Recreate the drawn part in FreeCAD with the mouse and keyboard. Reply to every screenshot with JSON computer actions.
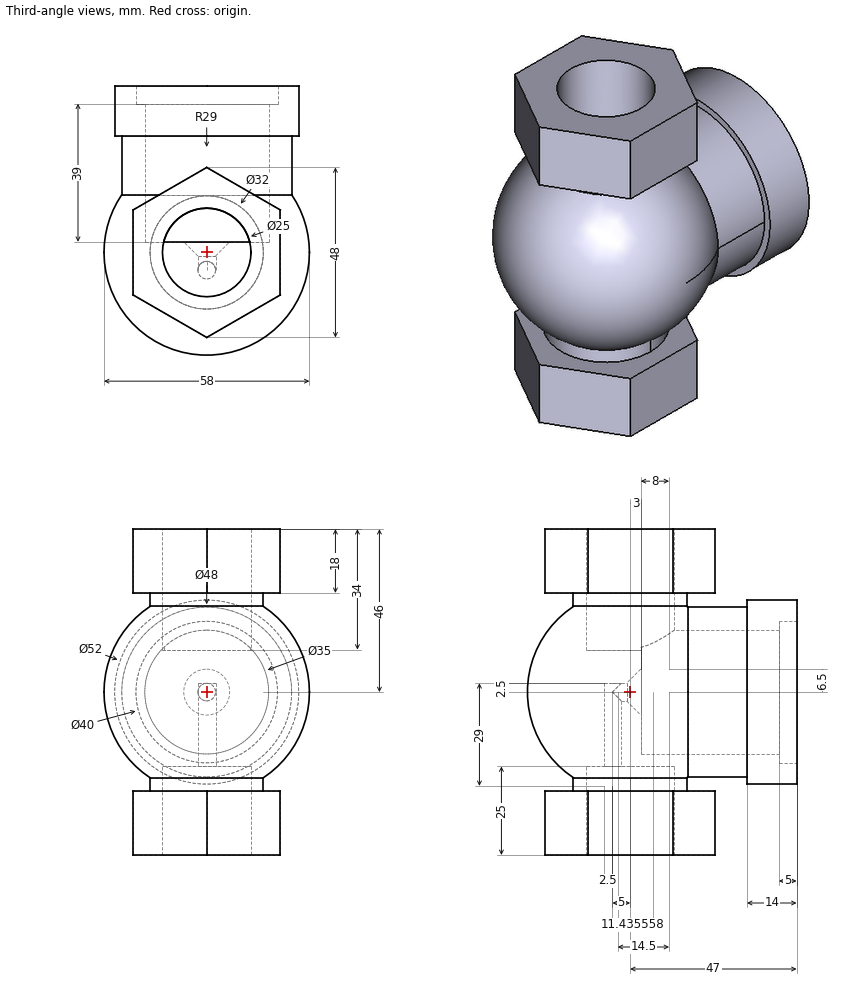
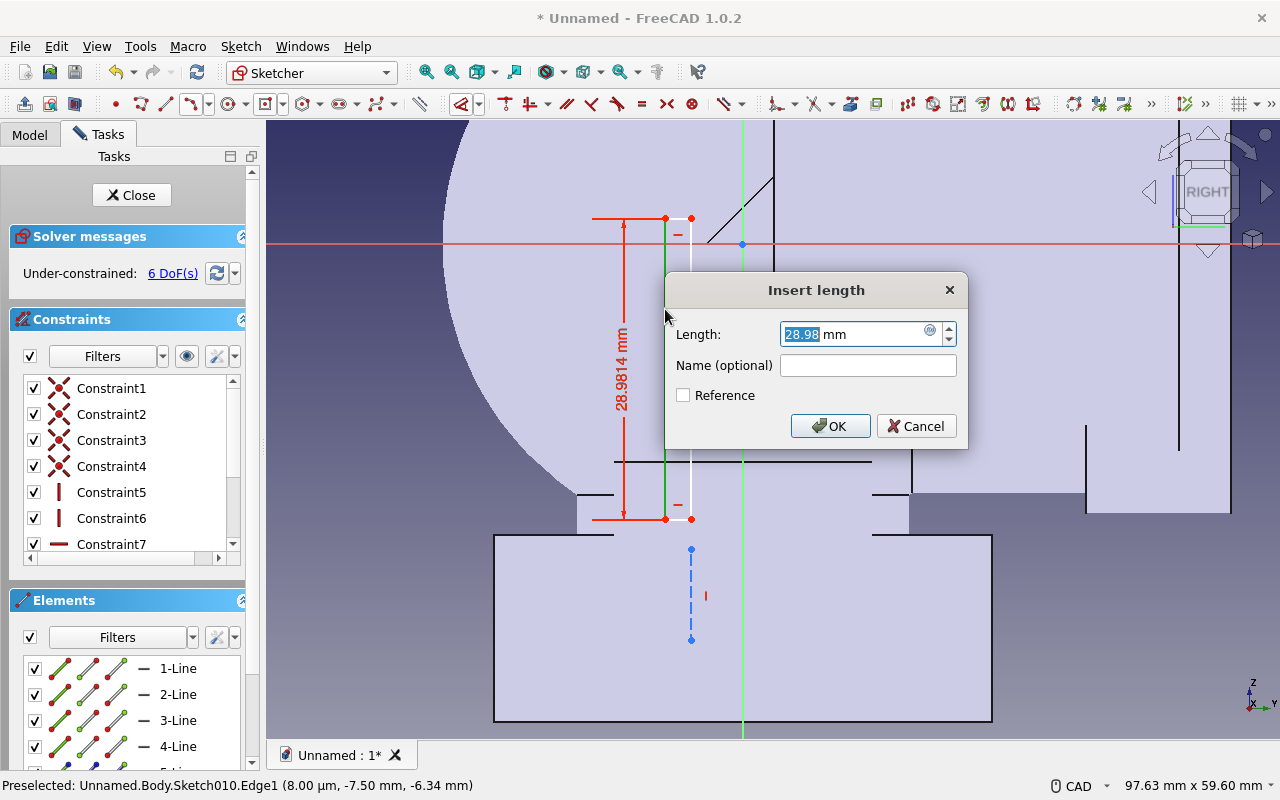
{"action": "type", "text": "29"}
{"action": "key", "text": "Return"}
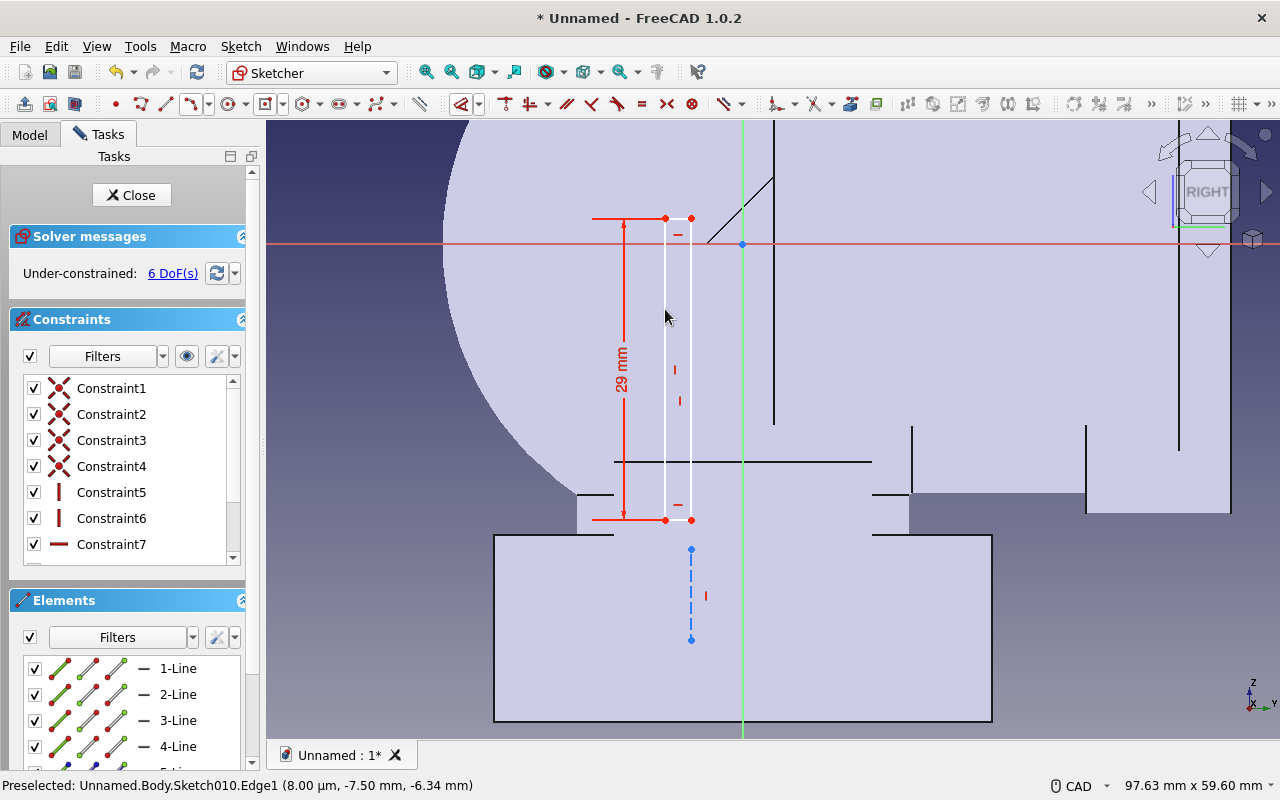
{"action": "left_click", "coordinate": [691, 520]}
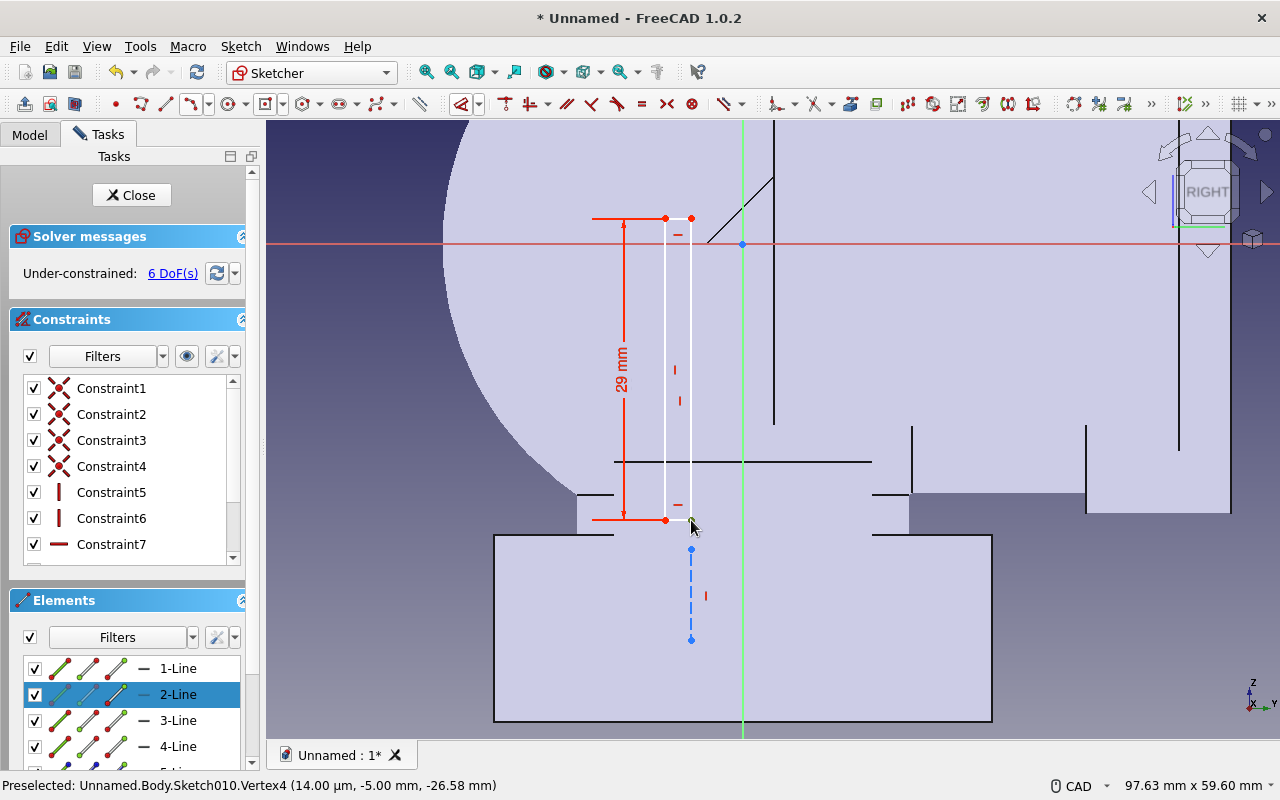
{"action": "key", "text": "l"}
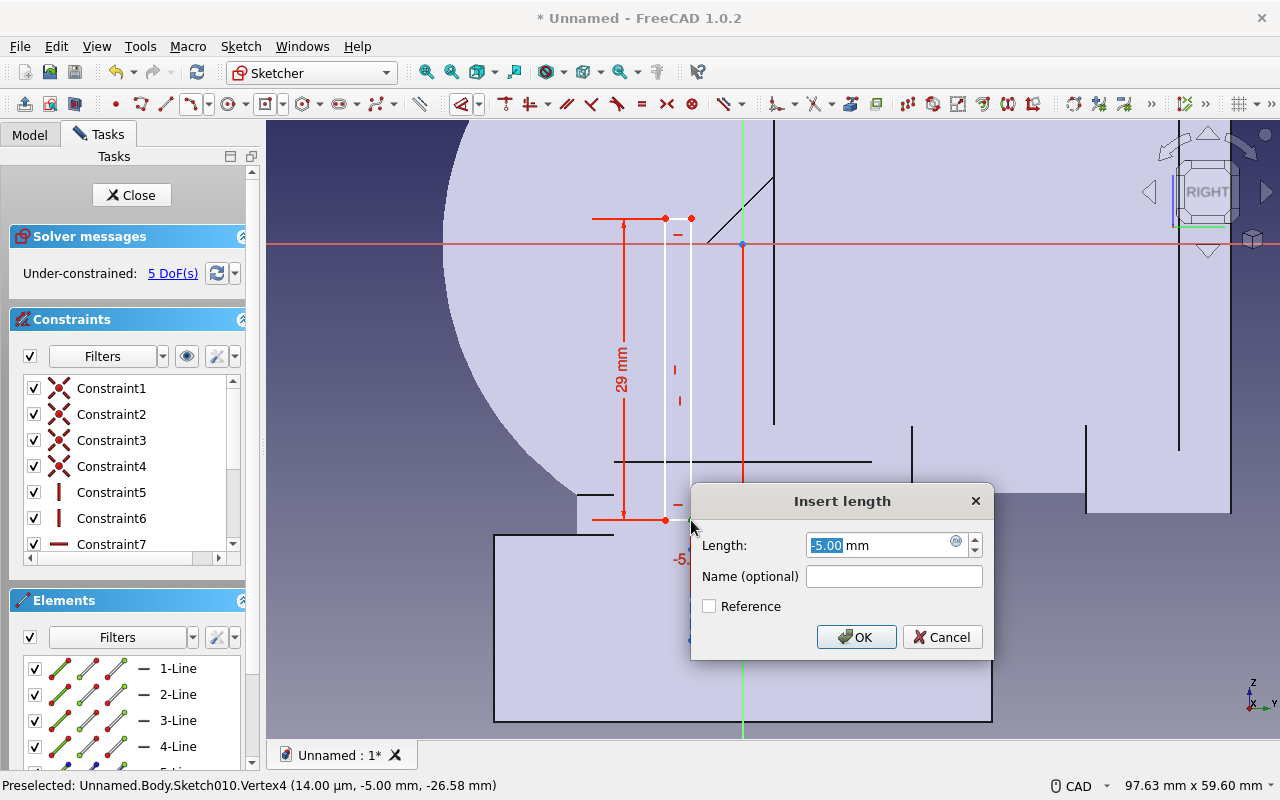
{"action": "type", "text": "-5"}
{"action": "key", "text": "Return"}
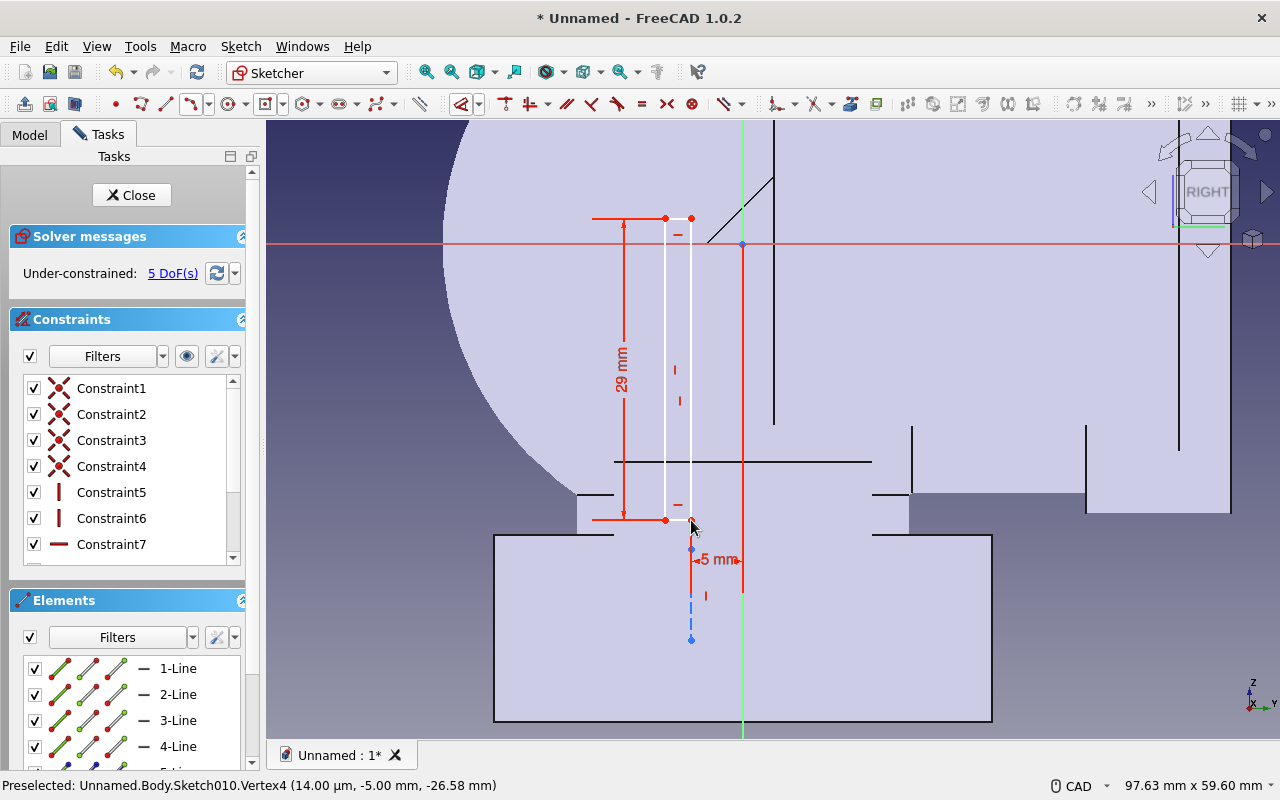
{"action": "left_click", "coordinate": [691, 550]}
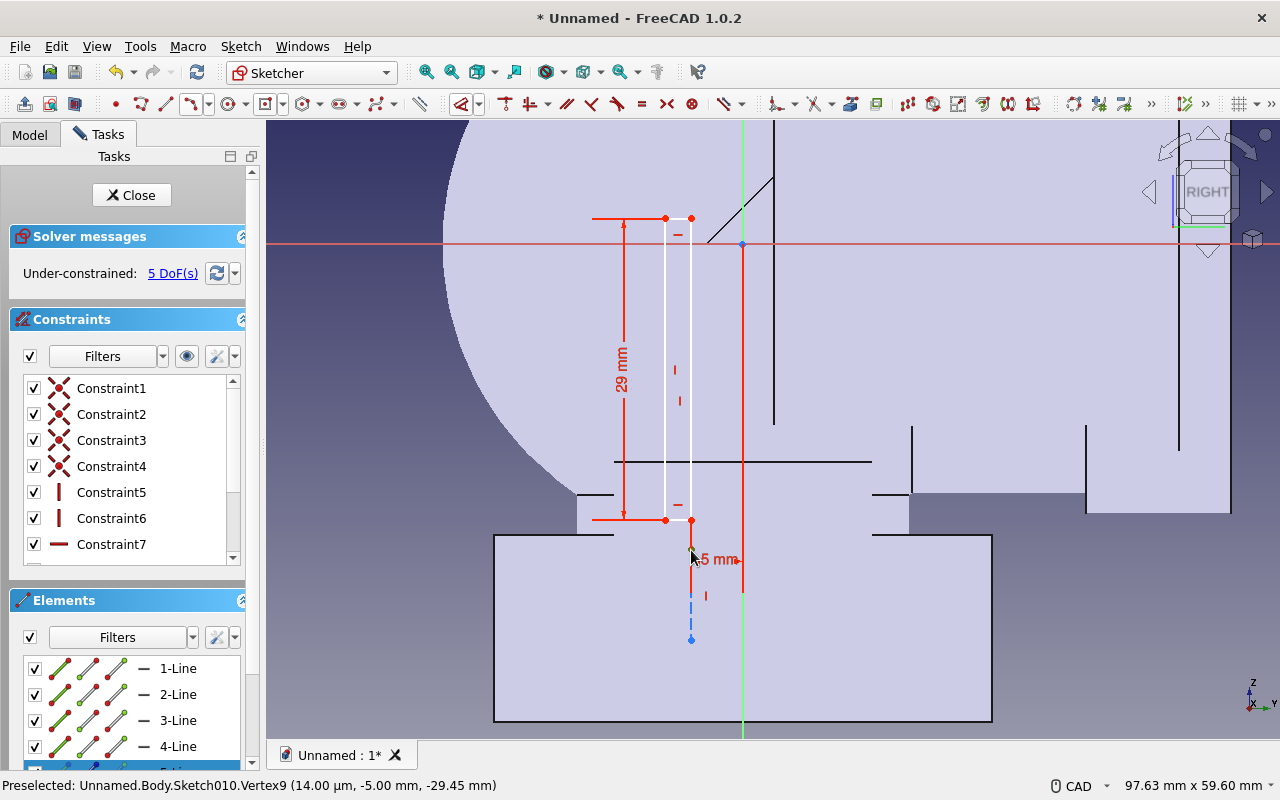
{"action": "key", "text": "l"}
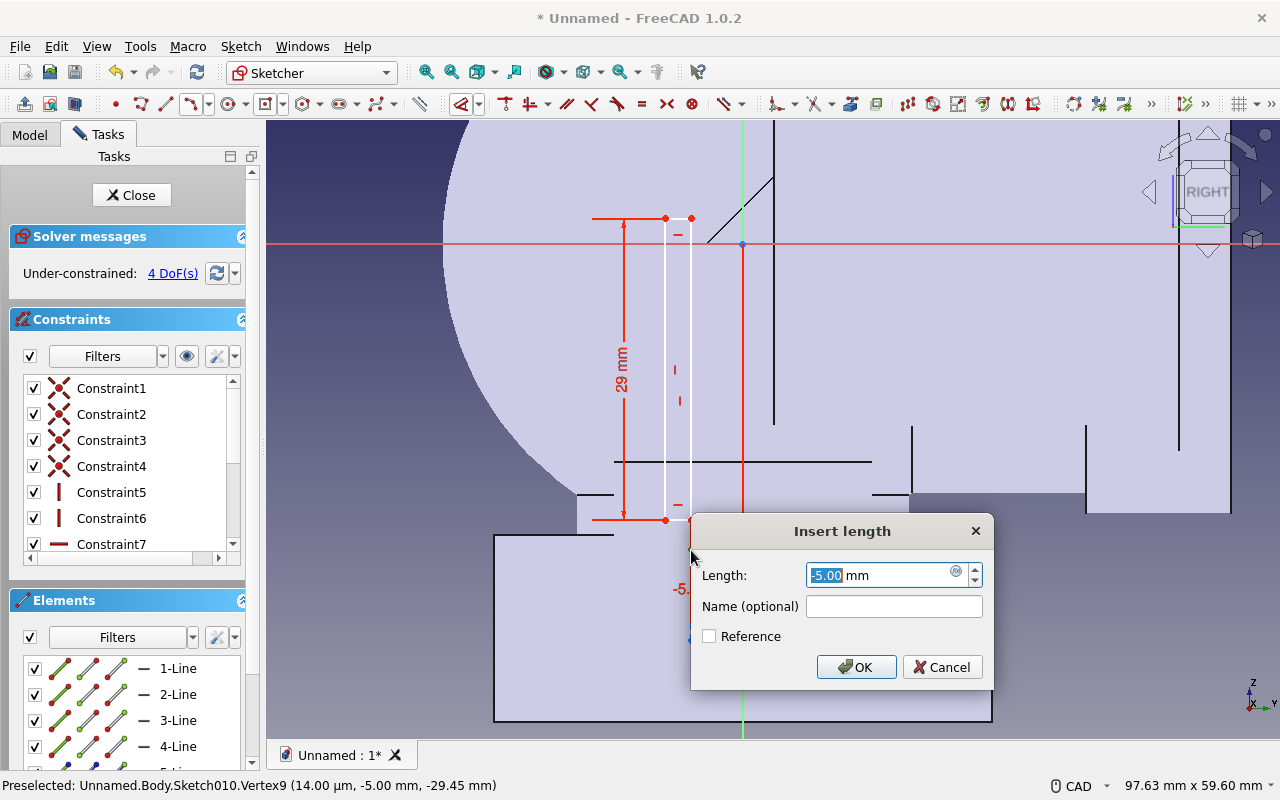
{"action": "type", "text": "-5"}
{"action": "key", "text": "Return"}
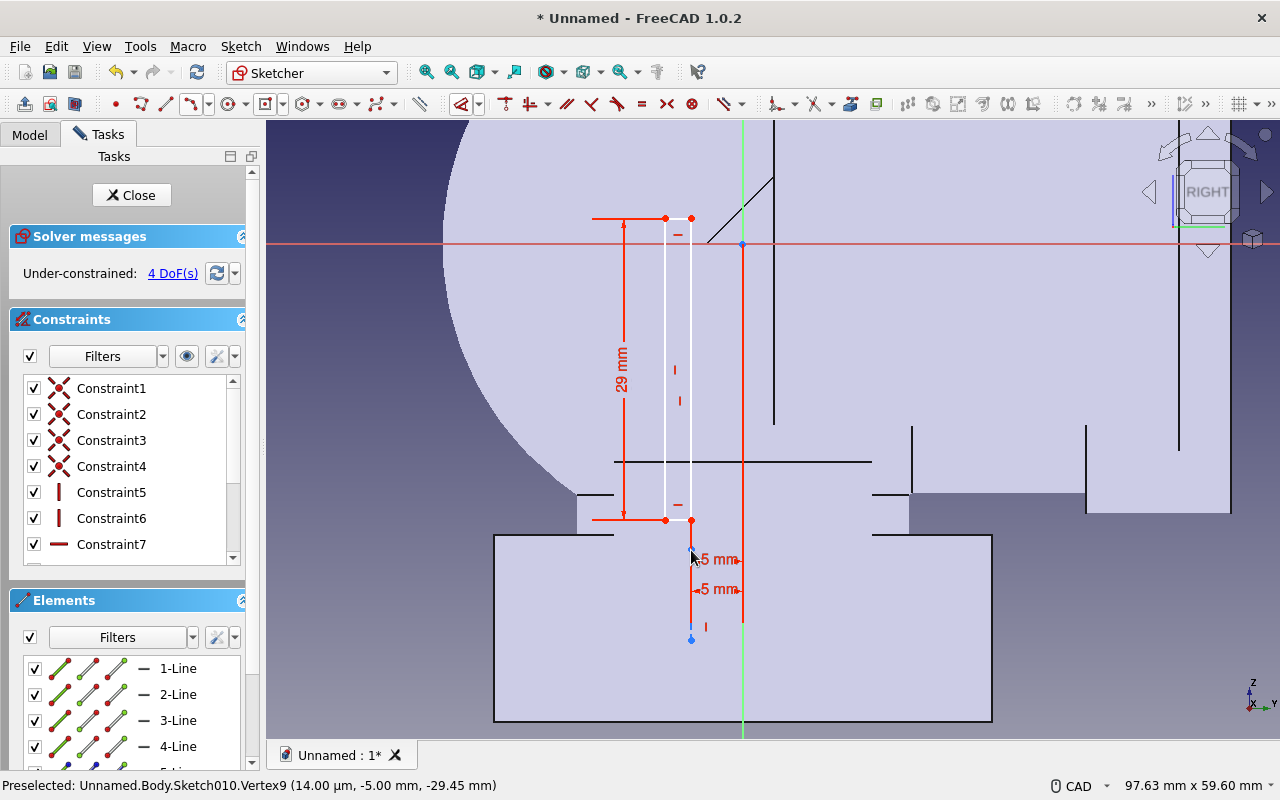
{"action": "scroll", "coordinate": [675, 520], "scroll_direction": "up", "scroll_amount": 3}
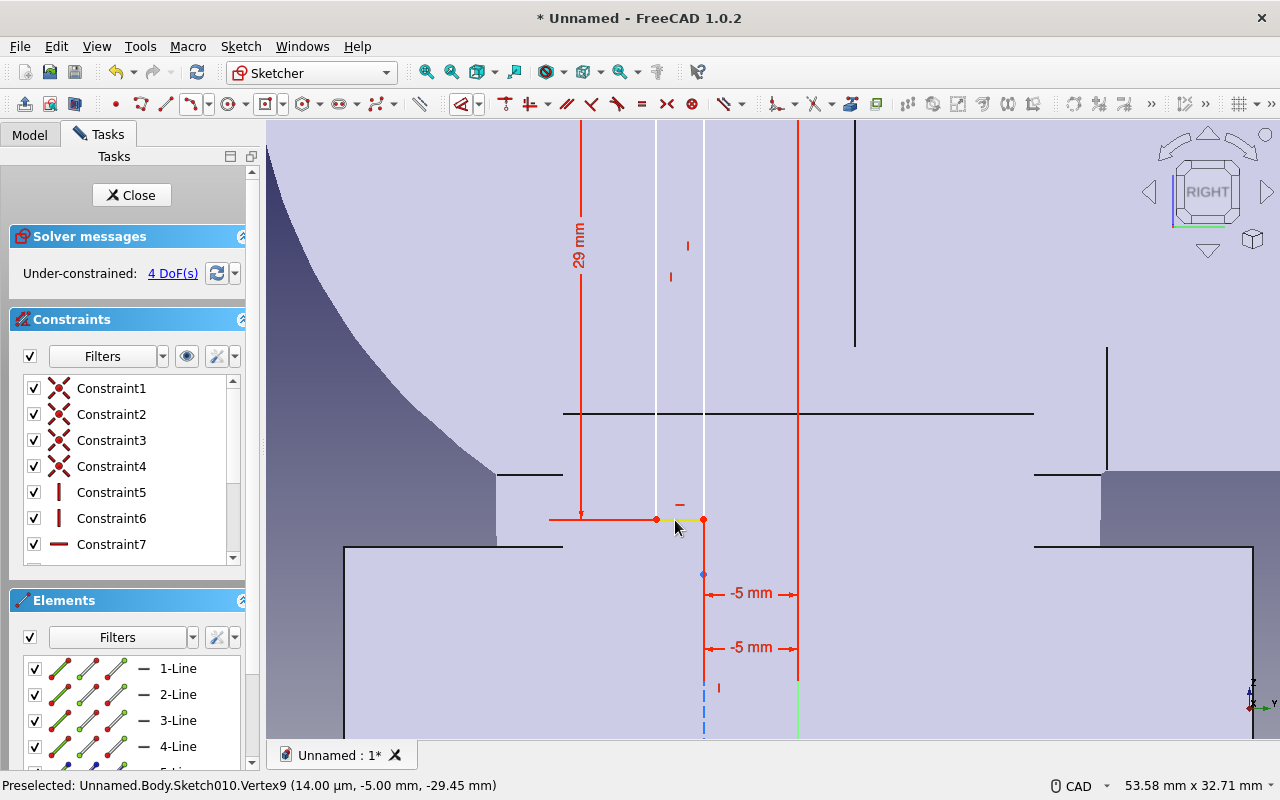
{"action": "left_click", "coordinate": [675, 520]}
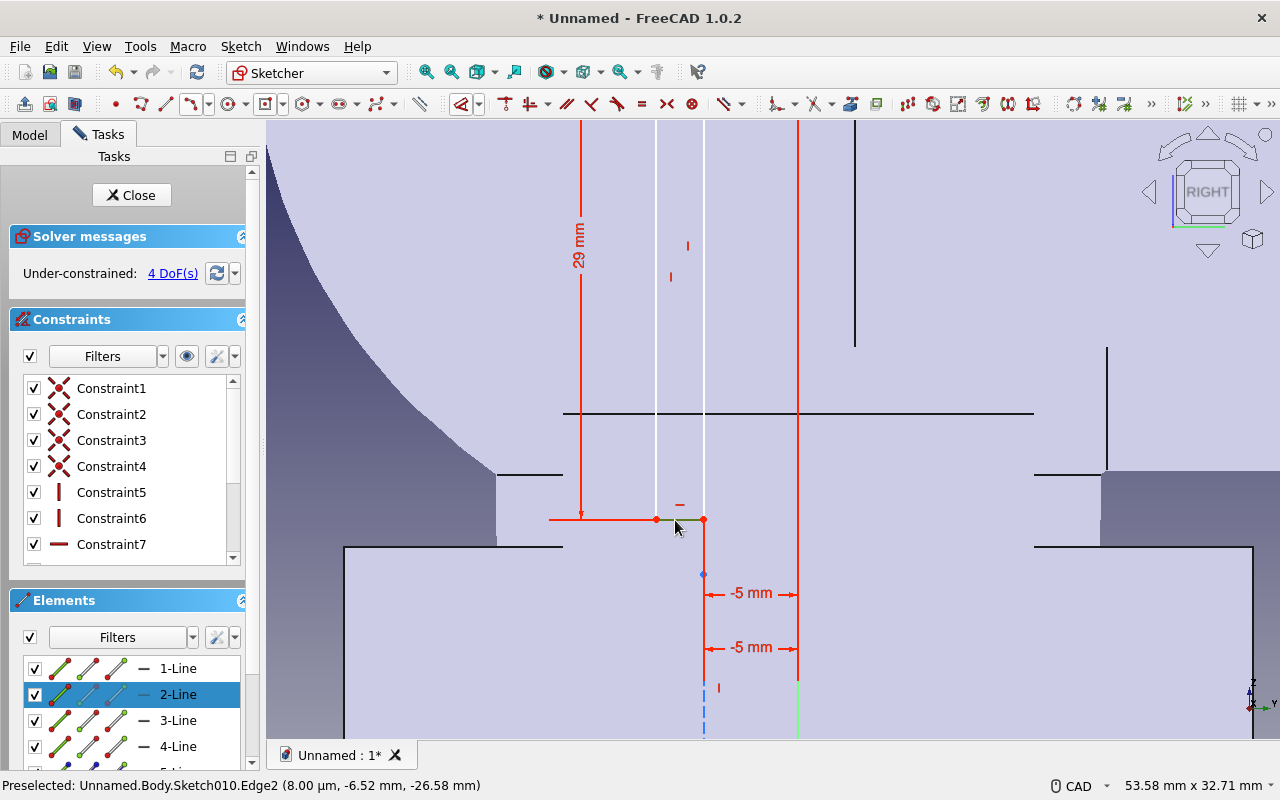
{"action": "left_click", "coordinate": [478, 104]}